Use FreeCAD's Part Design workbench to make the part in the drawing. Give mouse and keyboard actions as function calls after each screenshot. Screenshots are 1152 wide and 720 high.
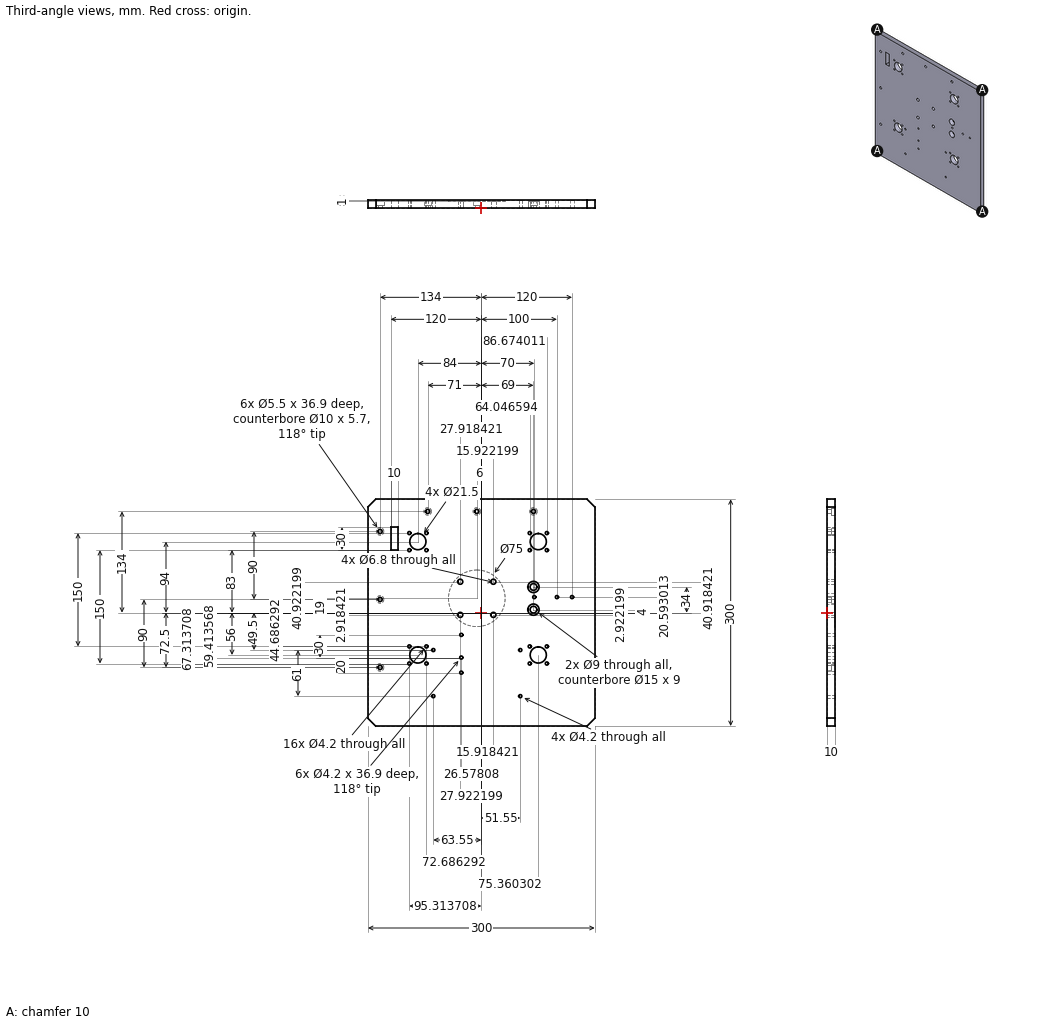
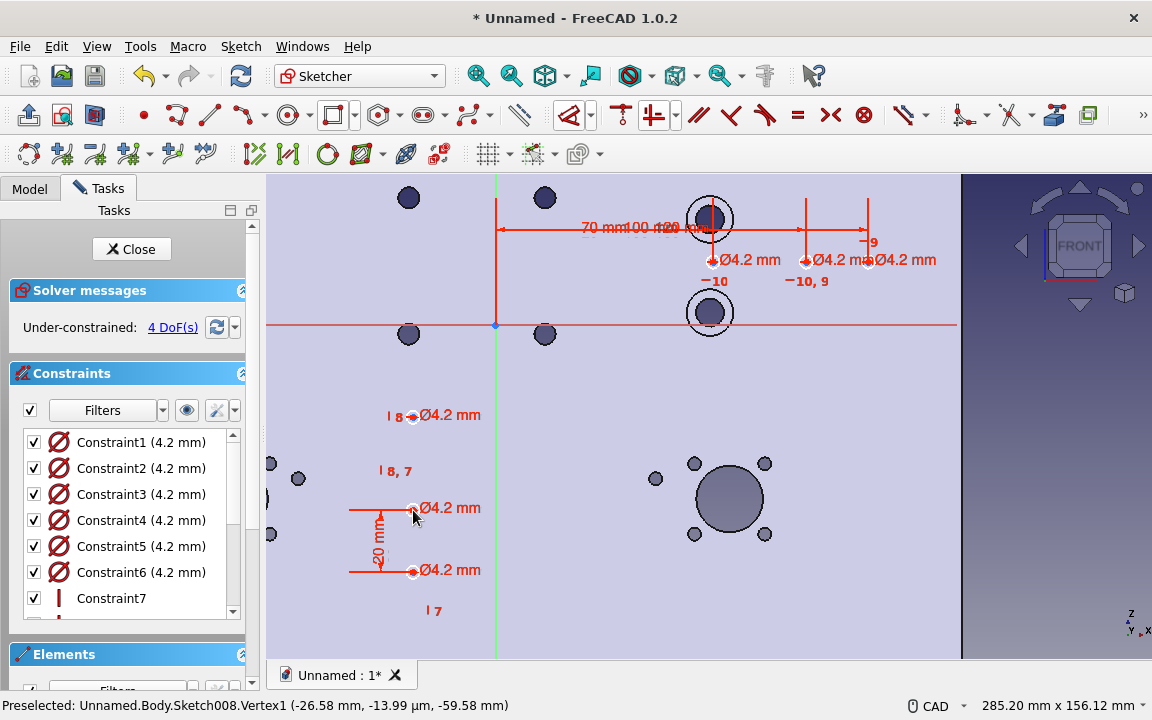
click(413, 417)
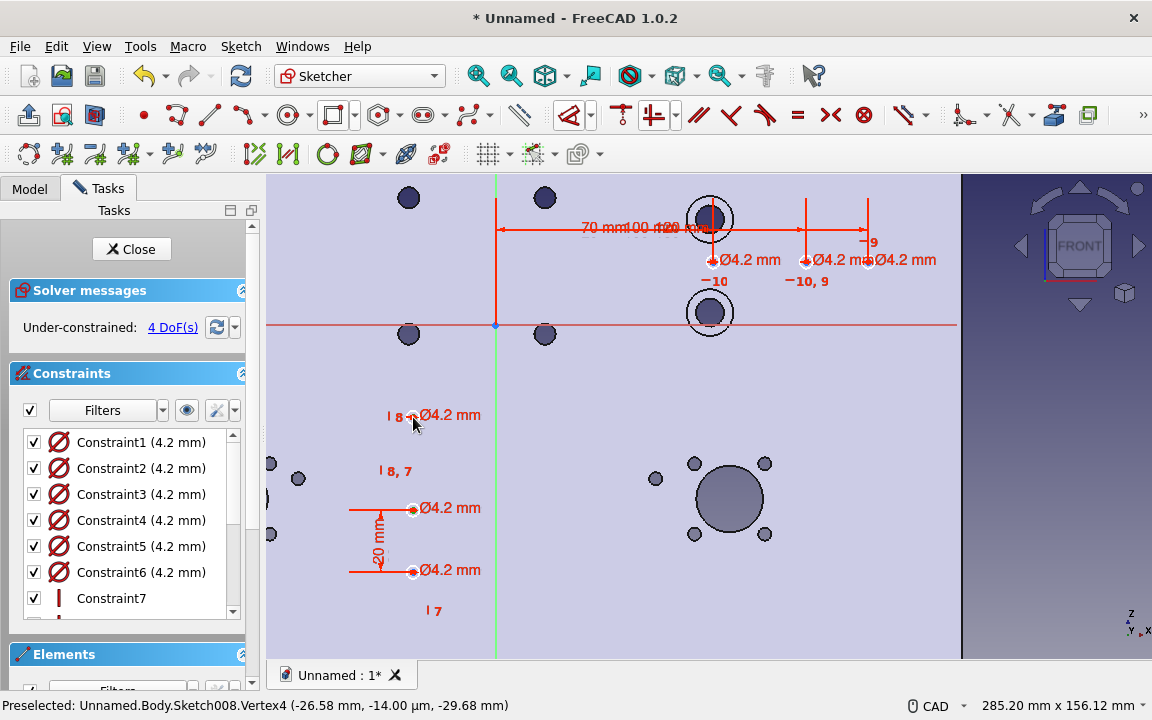
key(i)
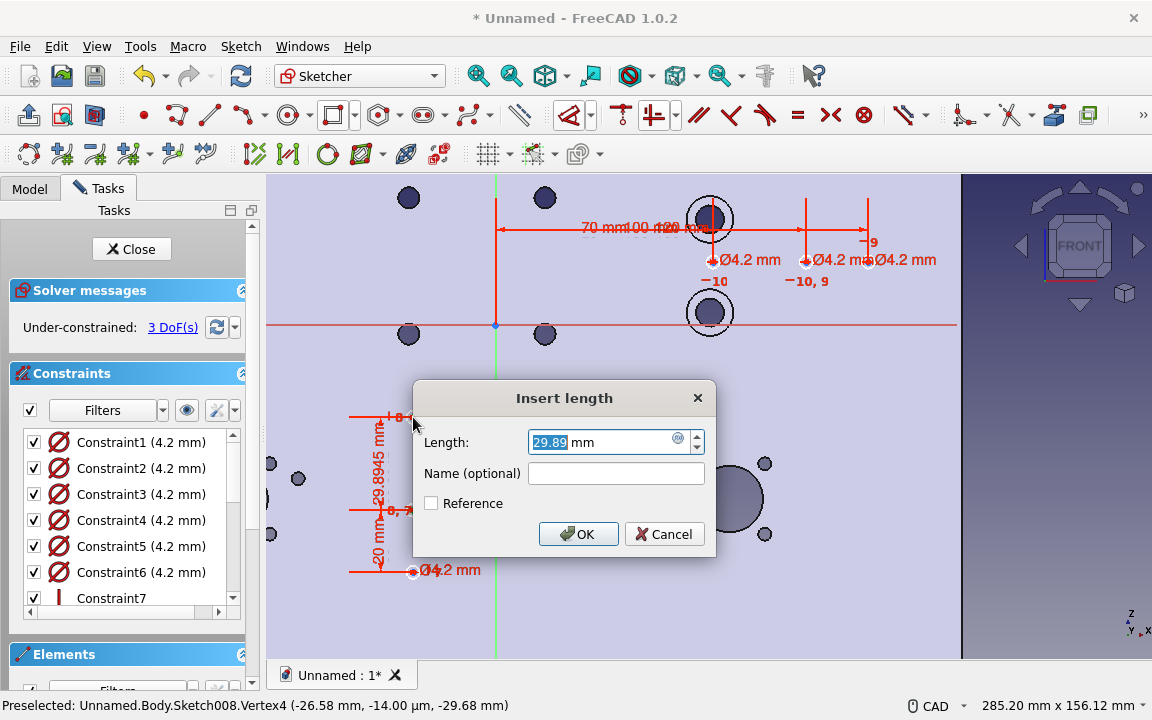
text(30)
key(Return)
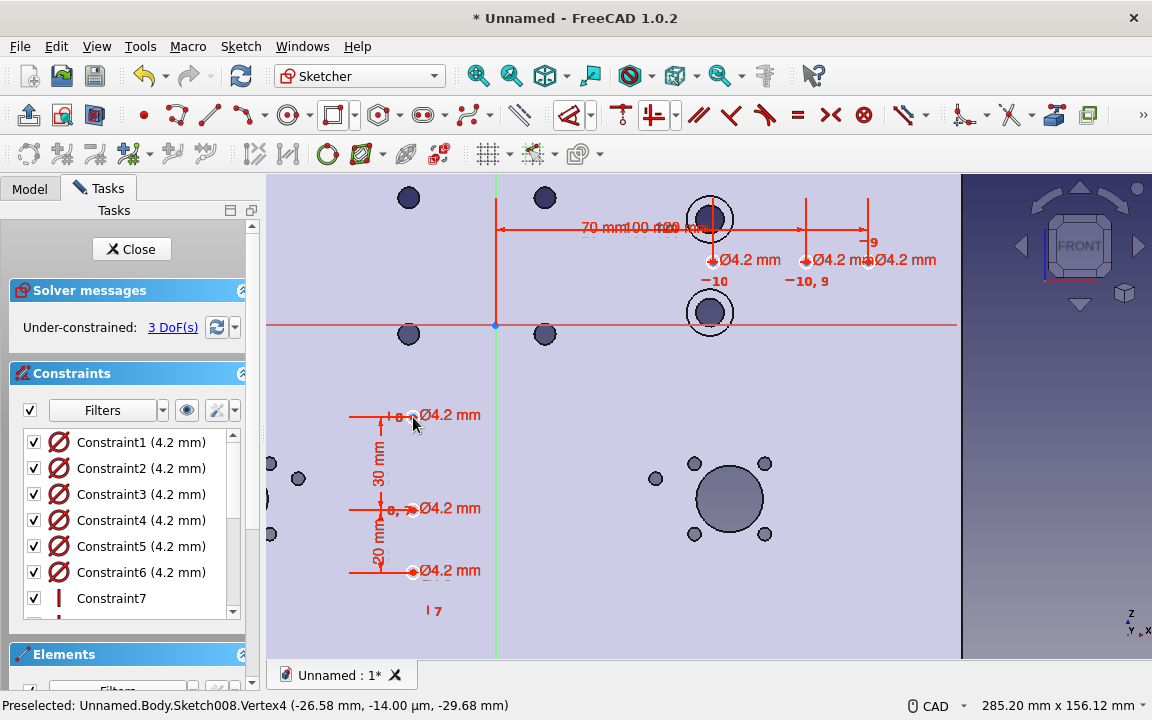
click(413, 510)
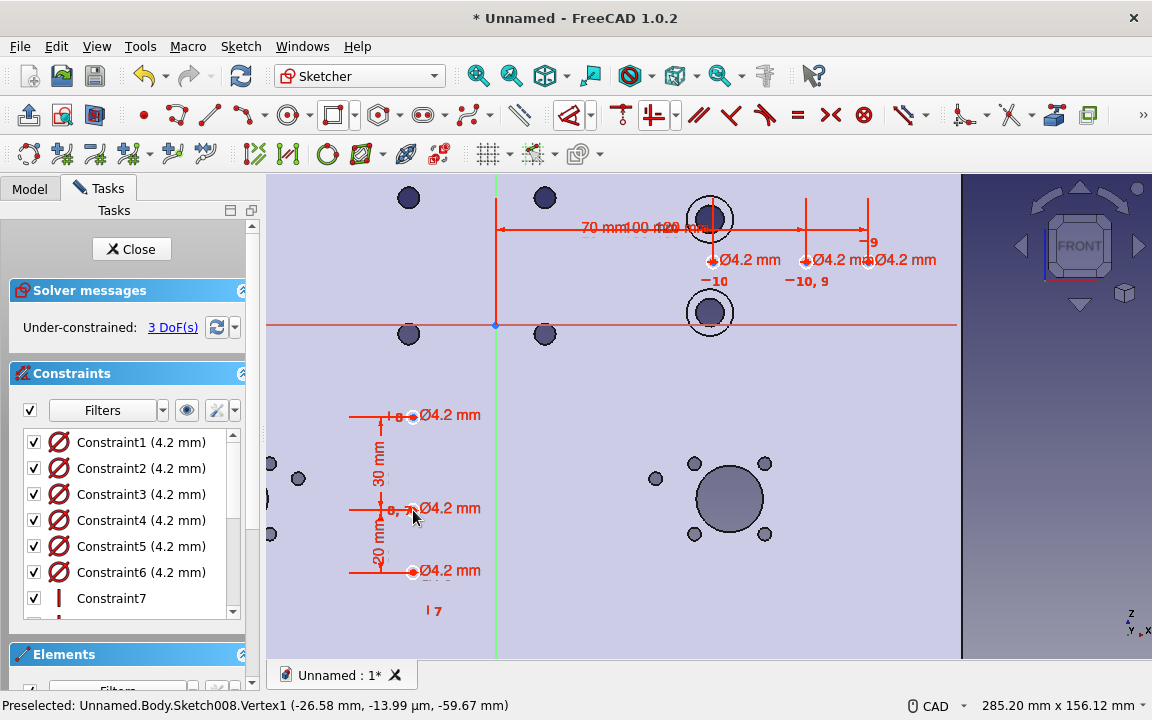
click(590, 116)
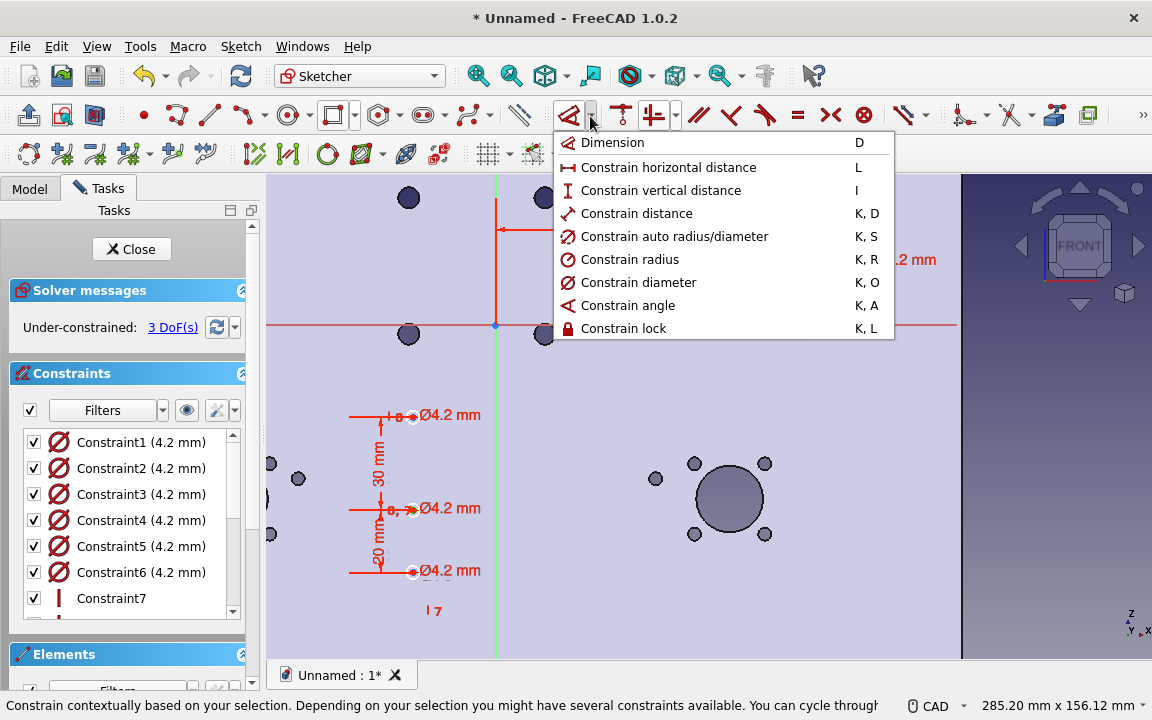
click(724, 168)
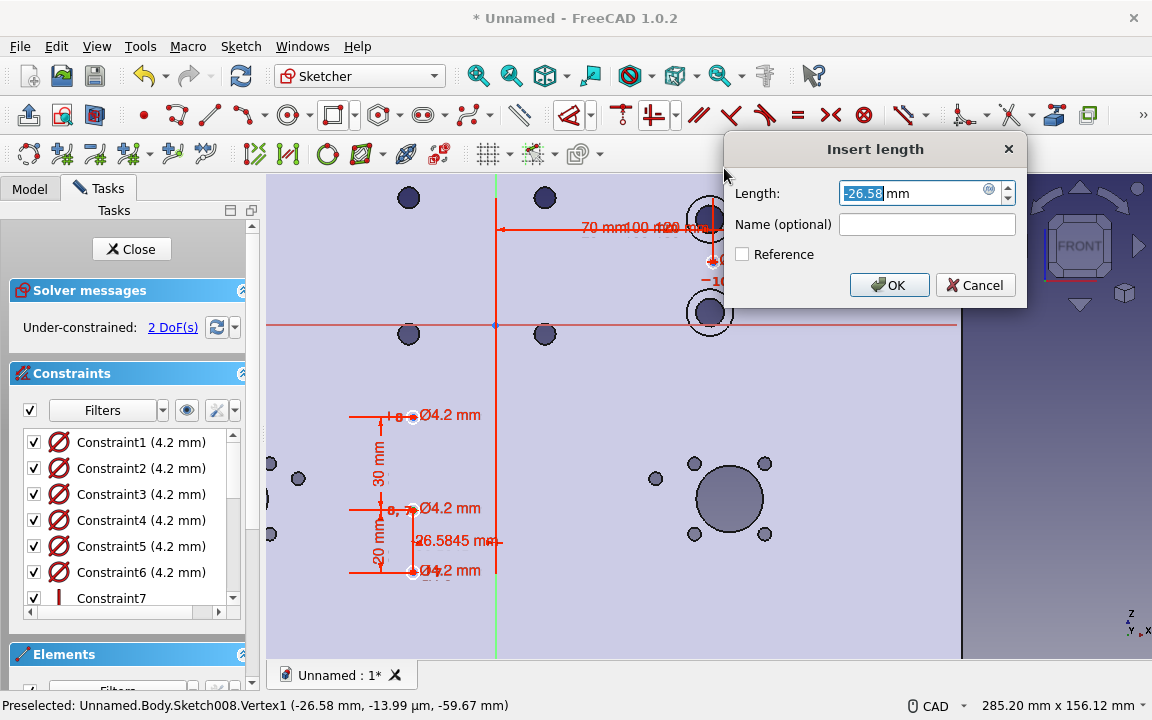
text(-26.57808)
key(Return)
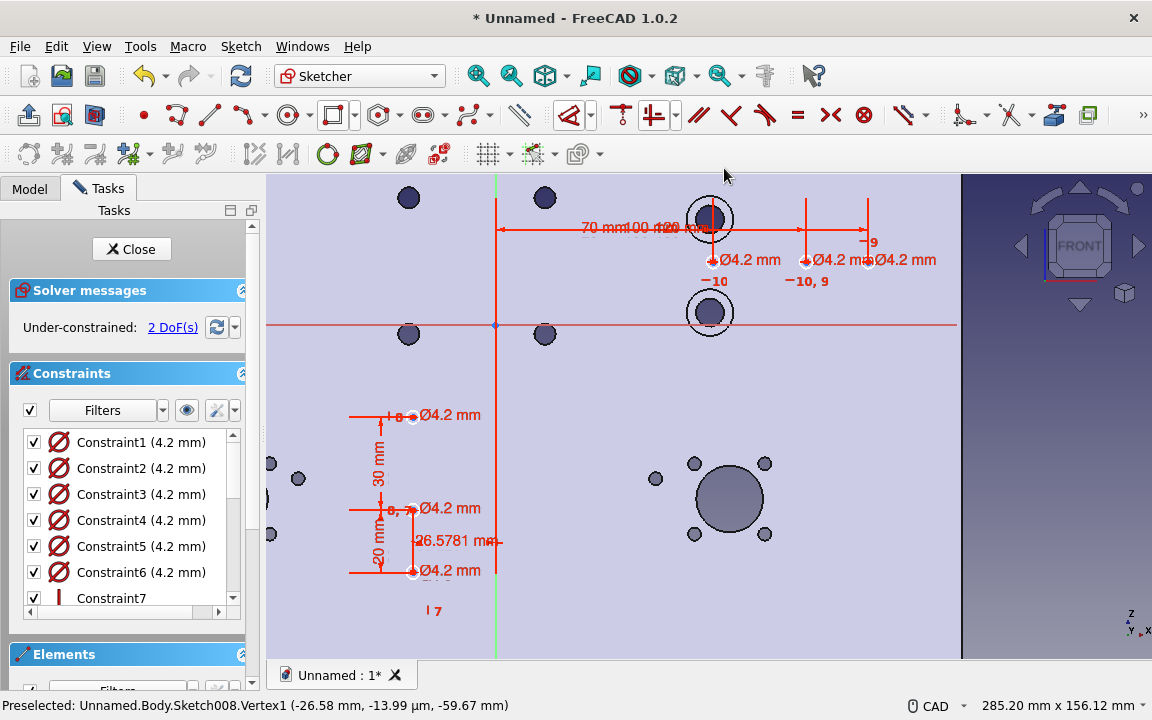
click(413, 510)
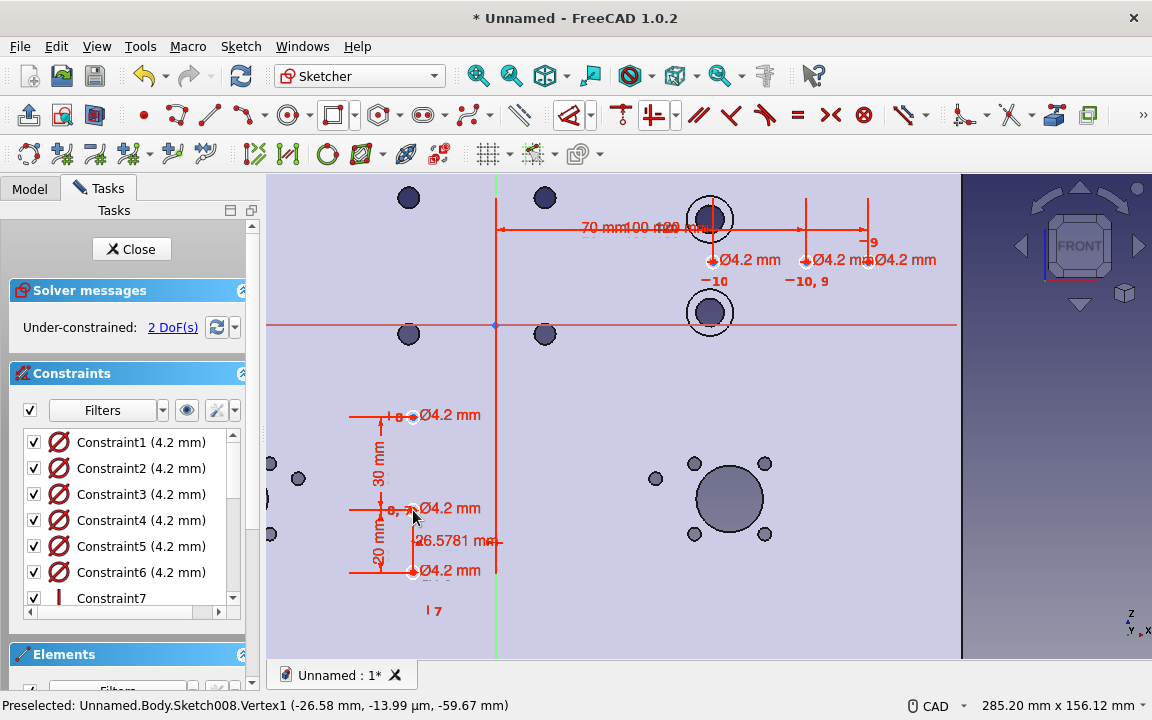
click(590, 116)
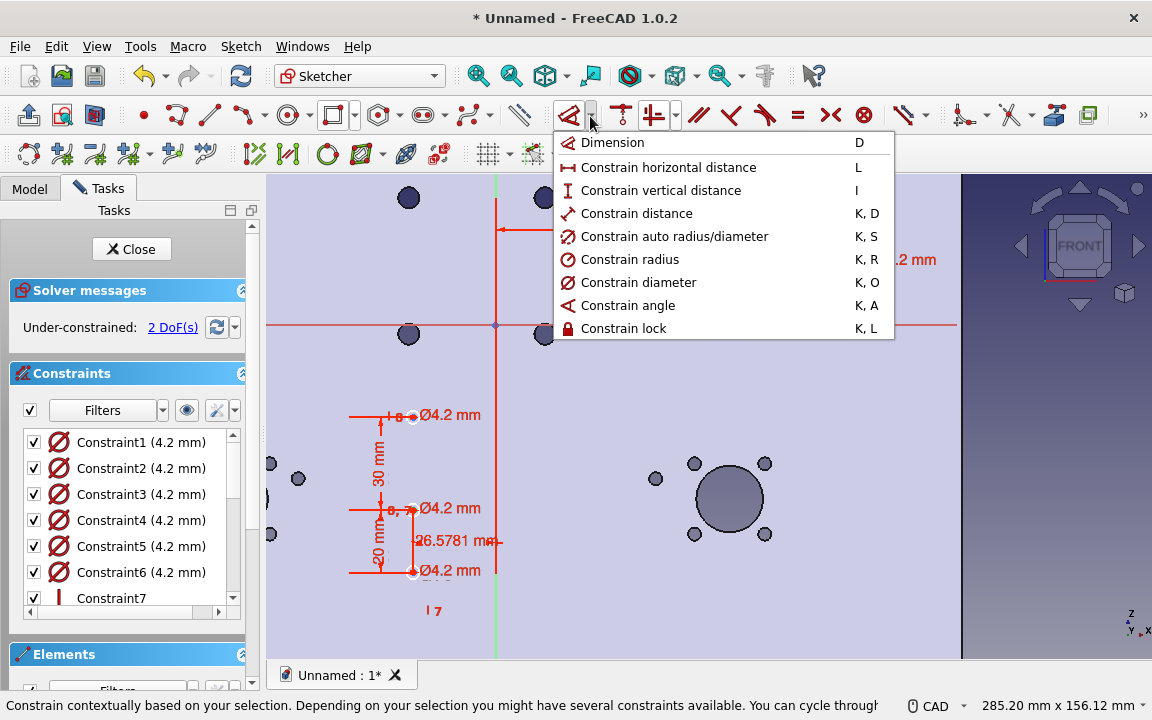
click(724, 190)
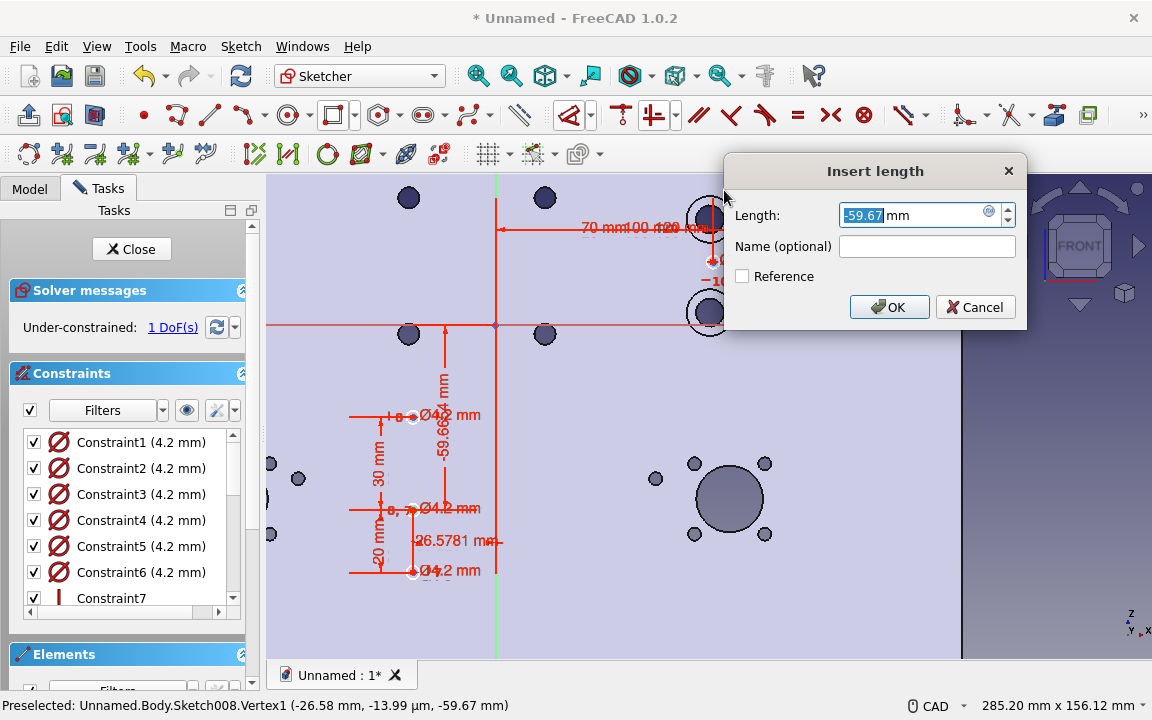
text(-59.413568)
key(Return)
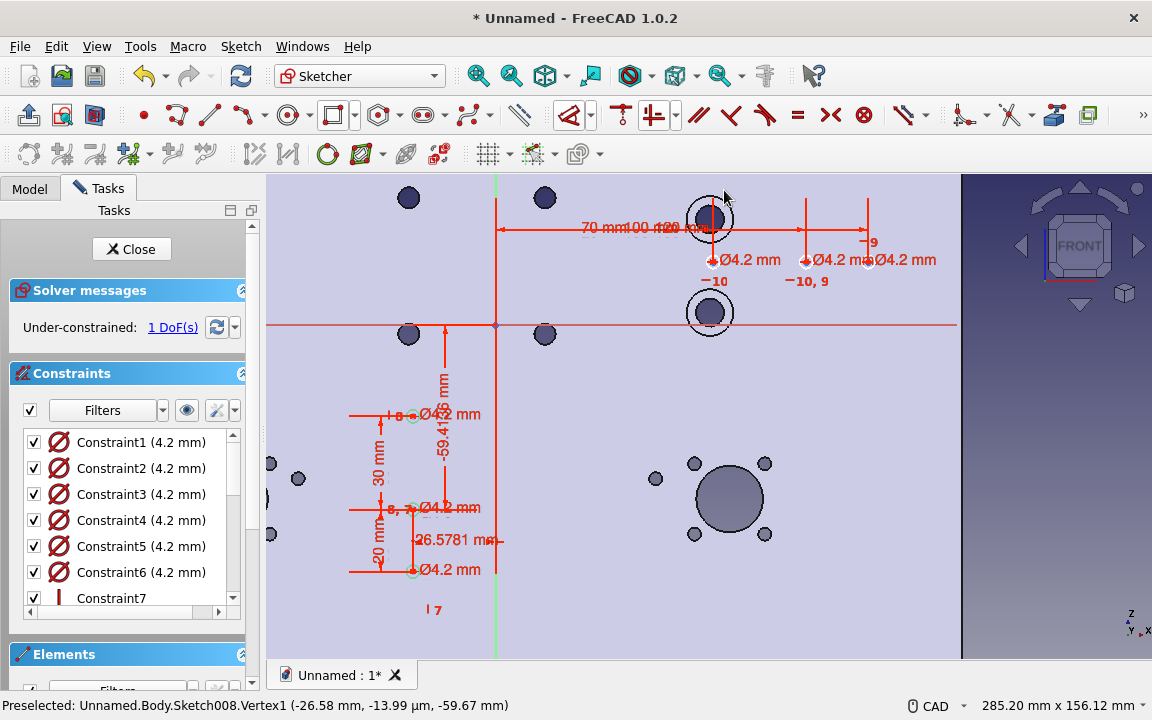
click(806, 262)